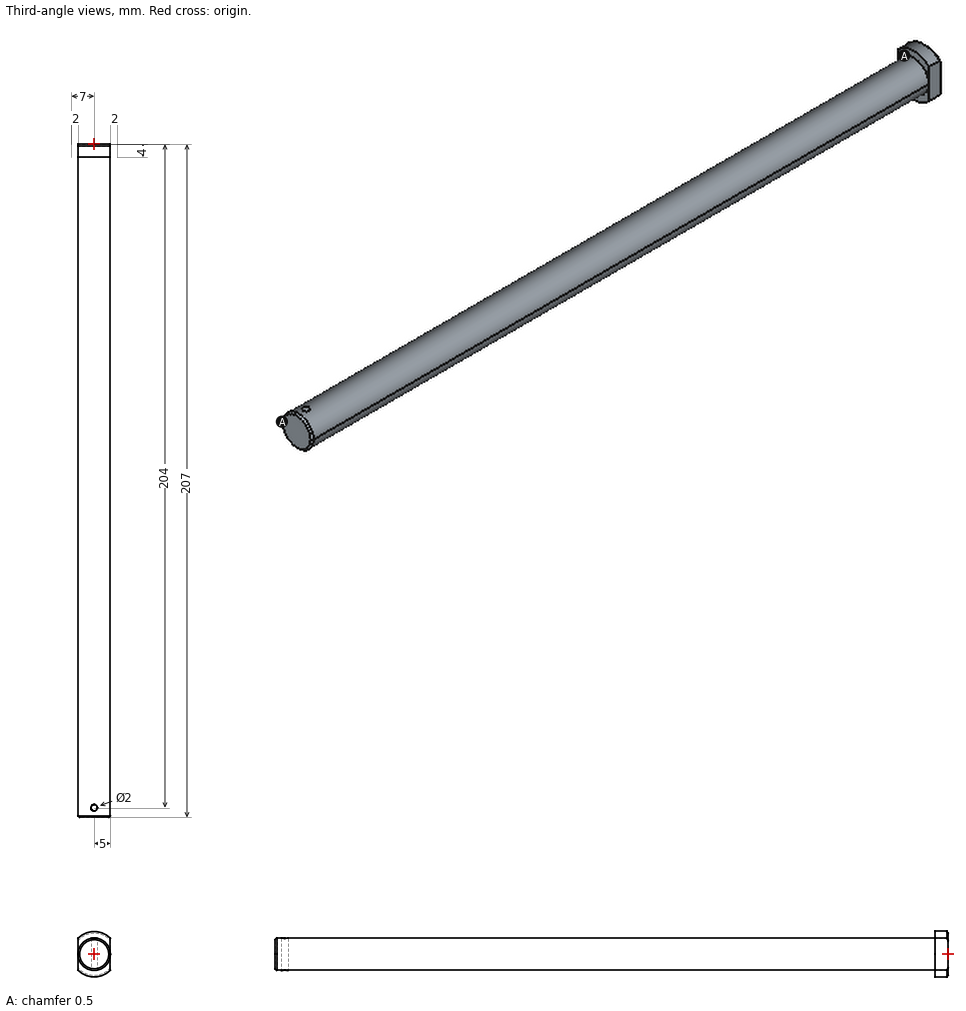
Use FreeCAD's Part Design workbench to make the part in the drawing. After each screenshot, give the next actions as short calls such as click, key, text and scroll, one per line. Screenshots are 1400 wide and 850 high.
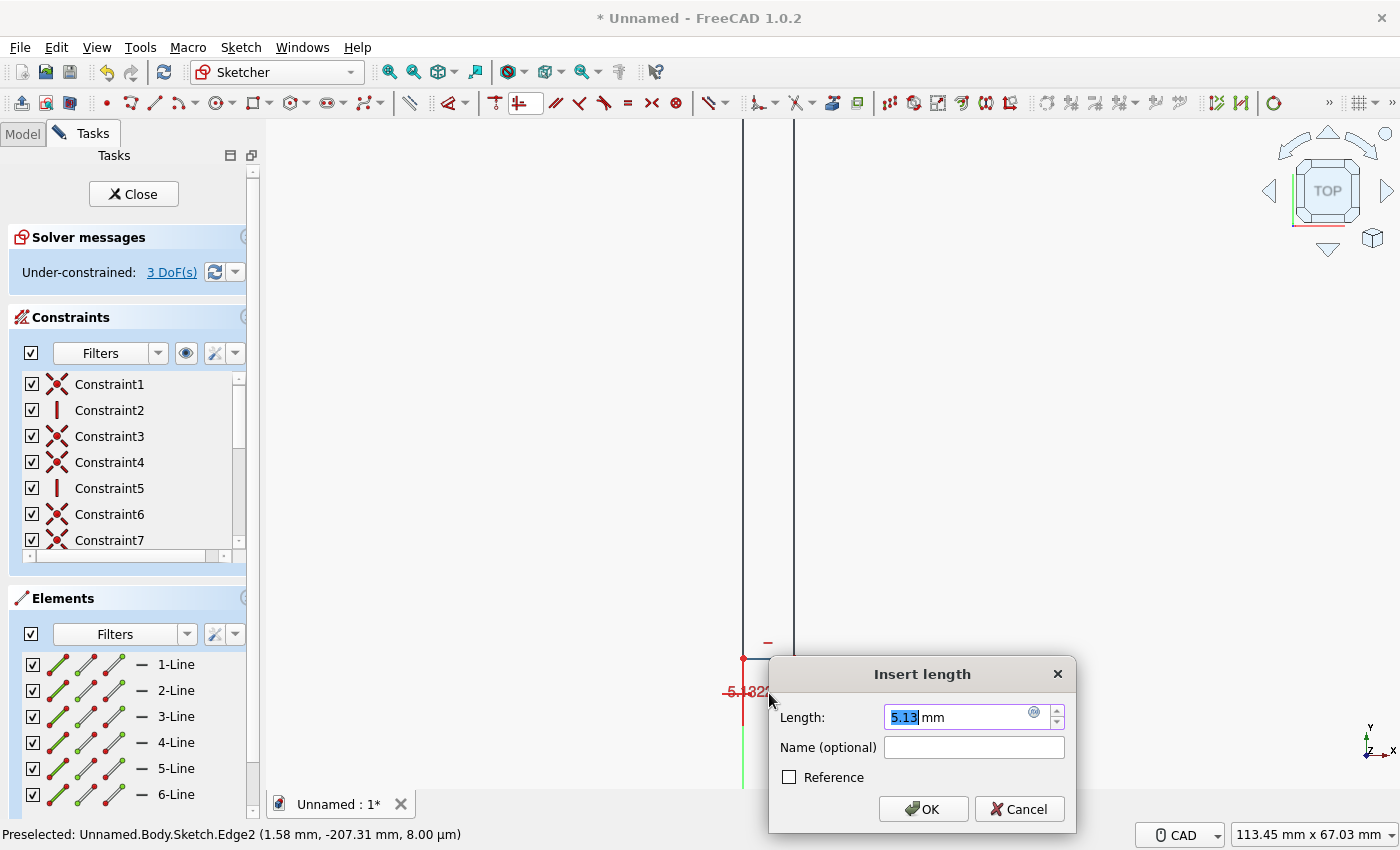
text(5)
key(Return)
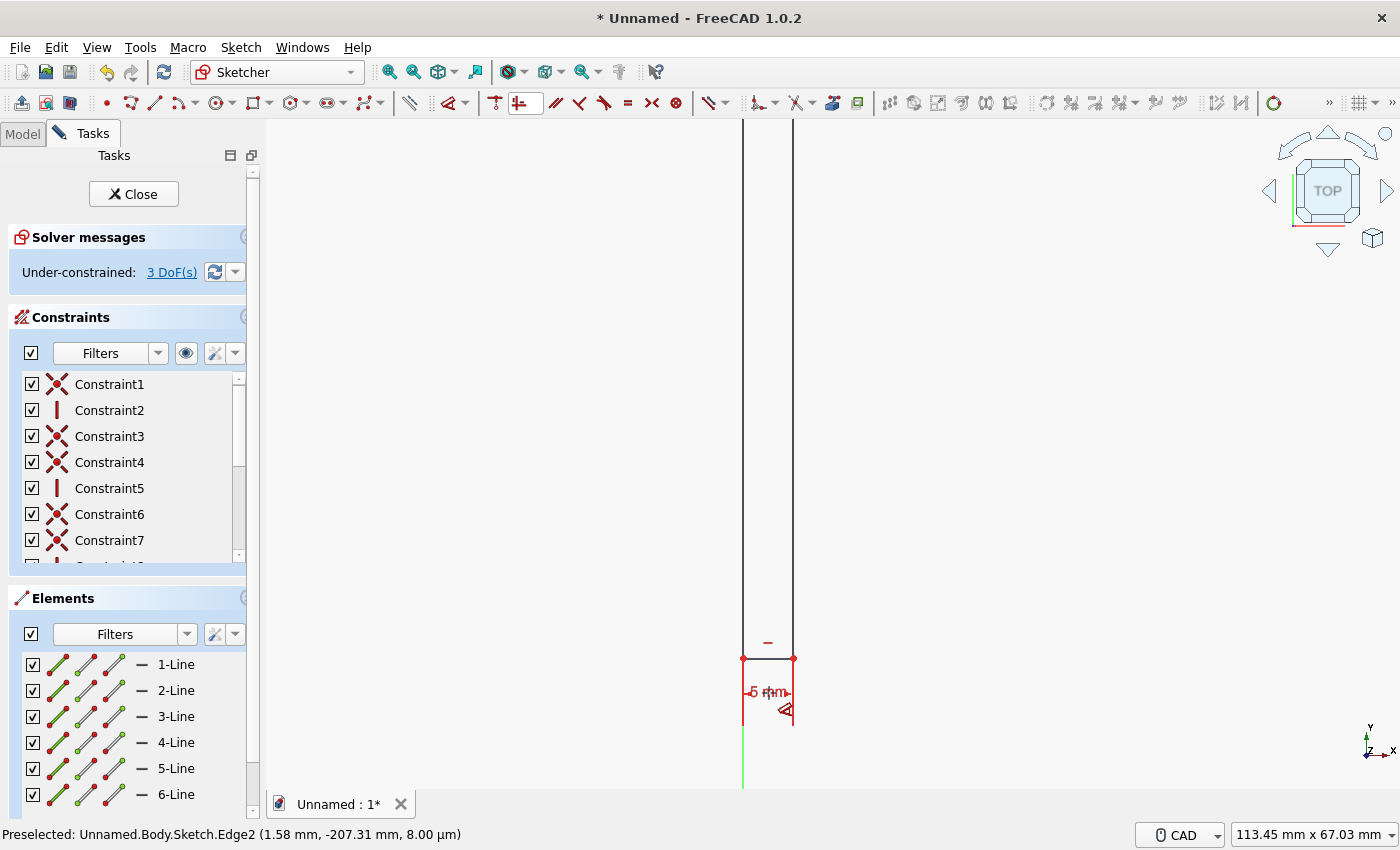
scroll(761, 665, down, 8)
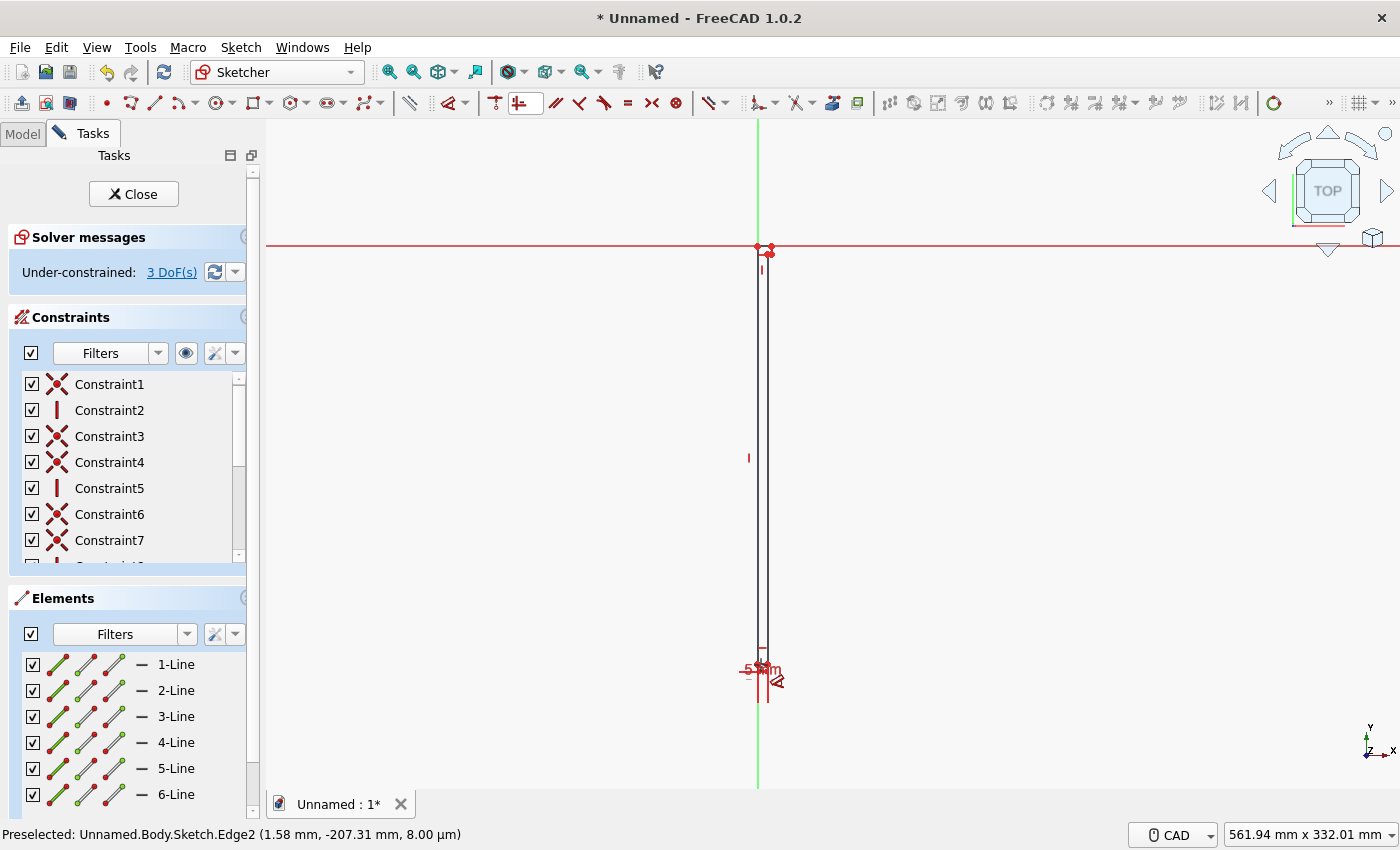
scroll(770, 255, up, 12)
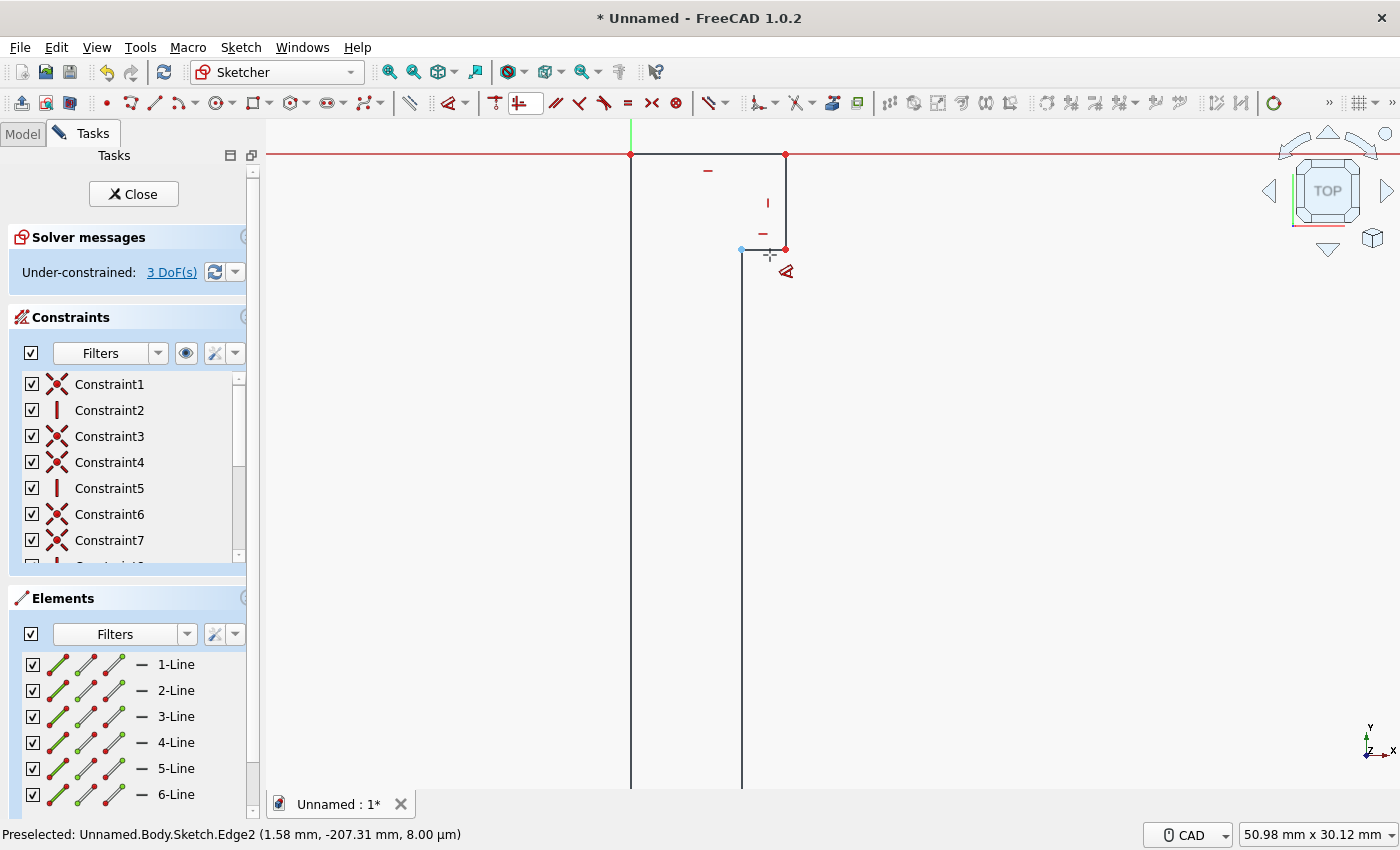
click(764, 250)
click(764, 216)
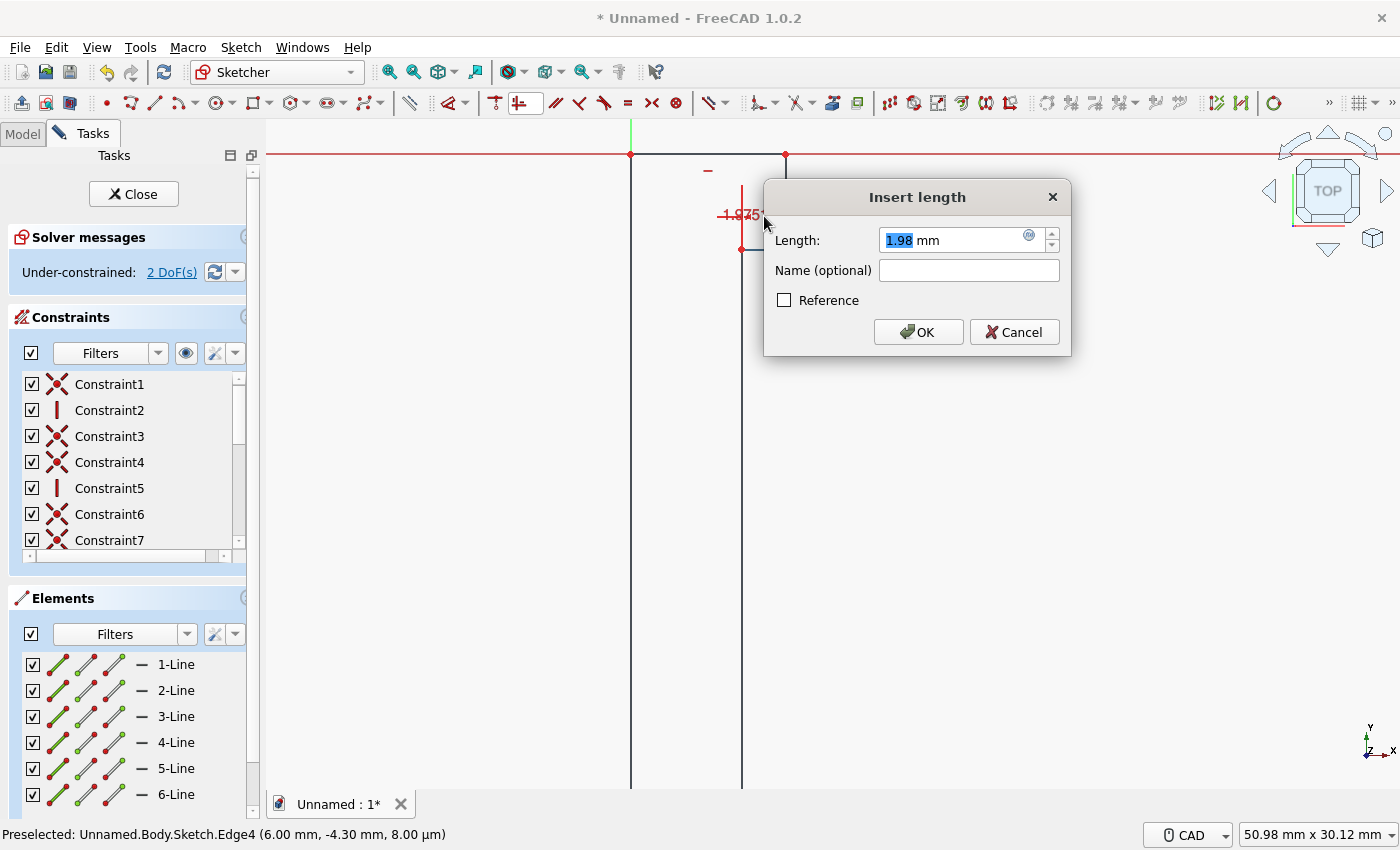
text(2)
key(Return)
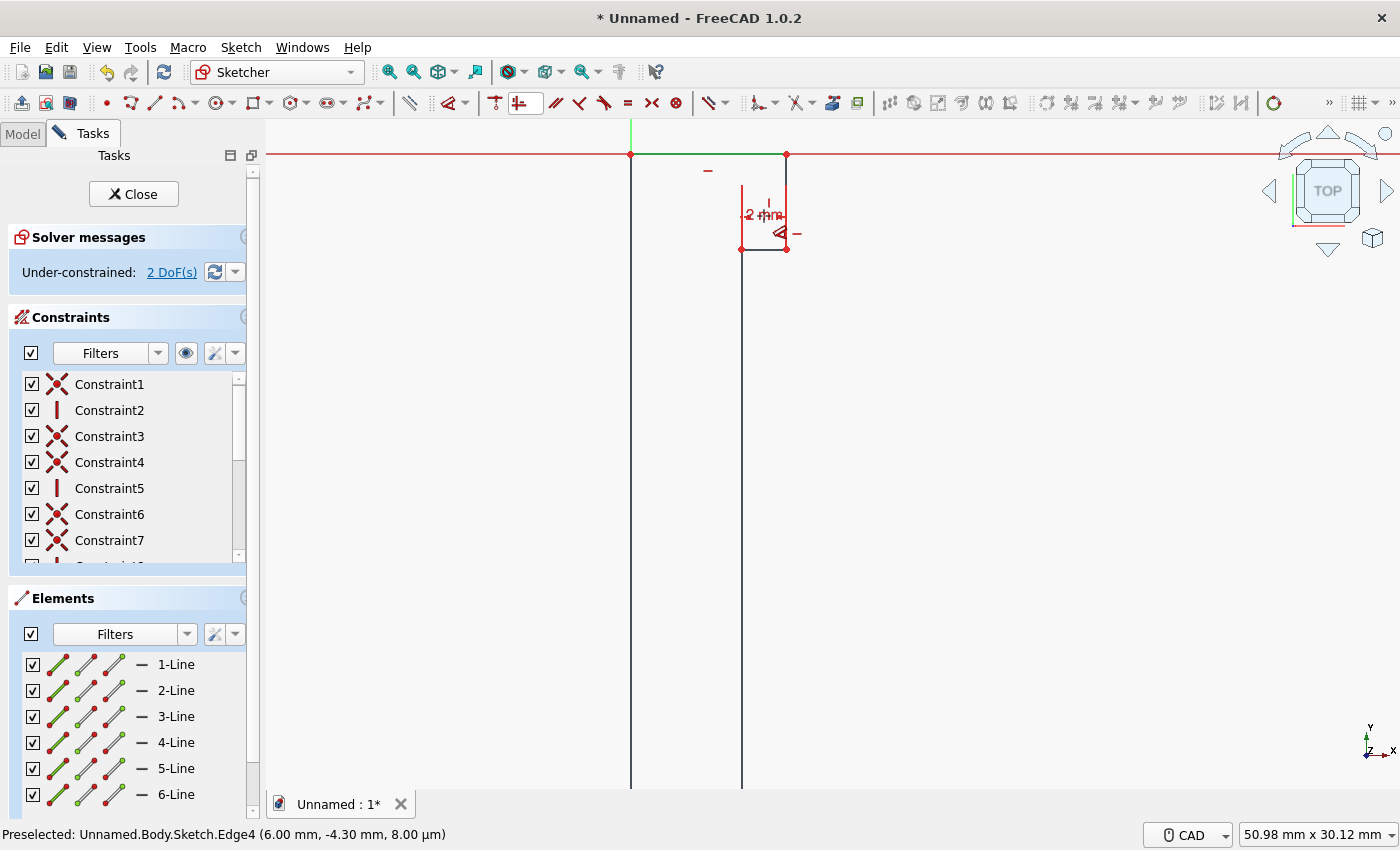
click(786, 221)
click(820, 180)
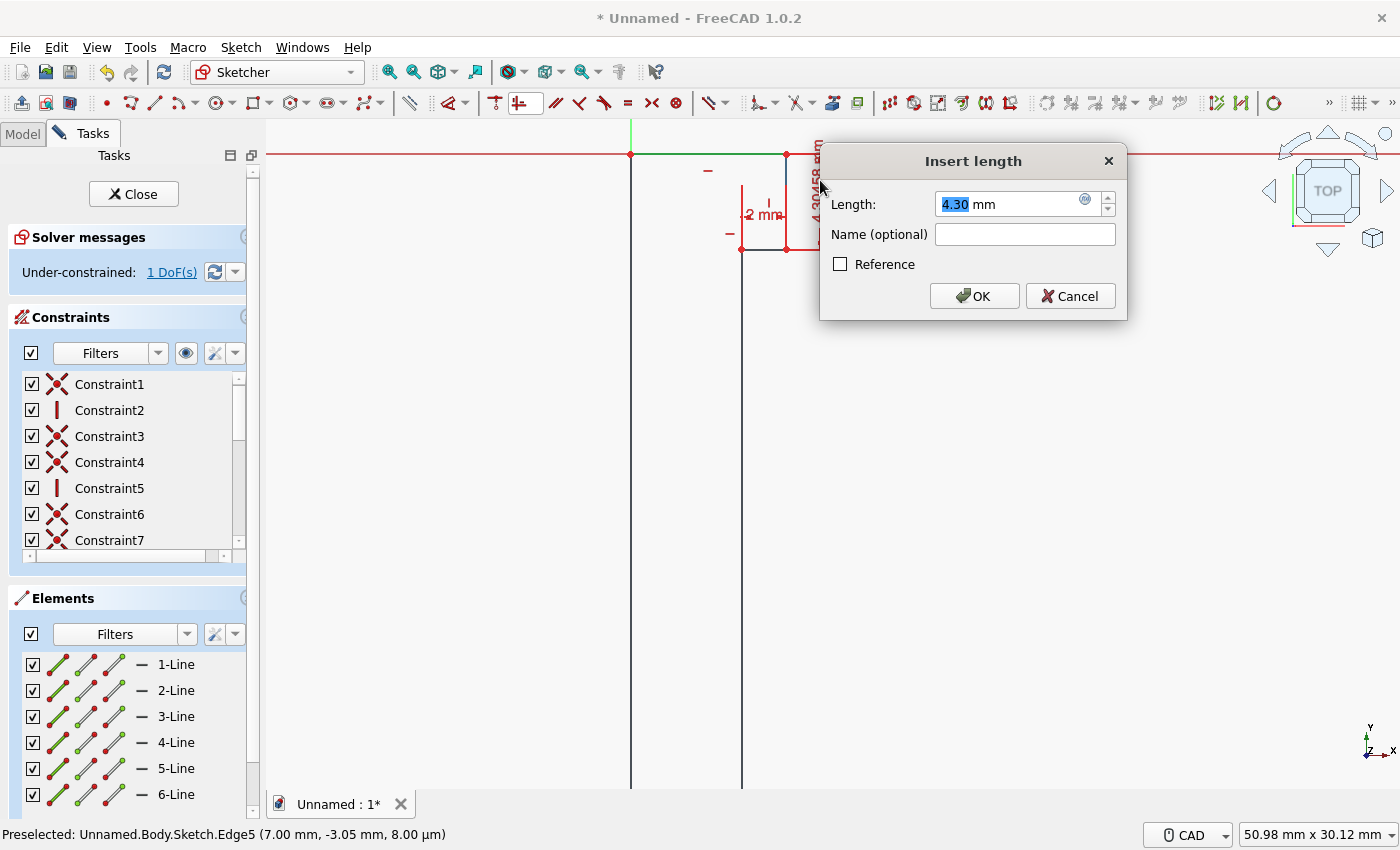
text(4)
key(Return)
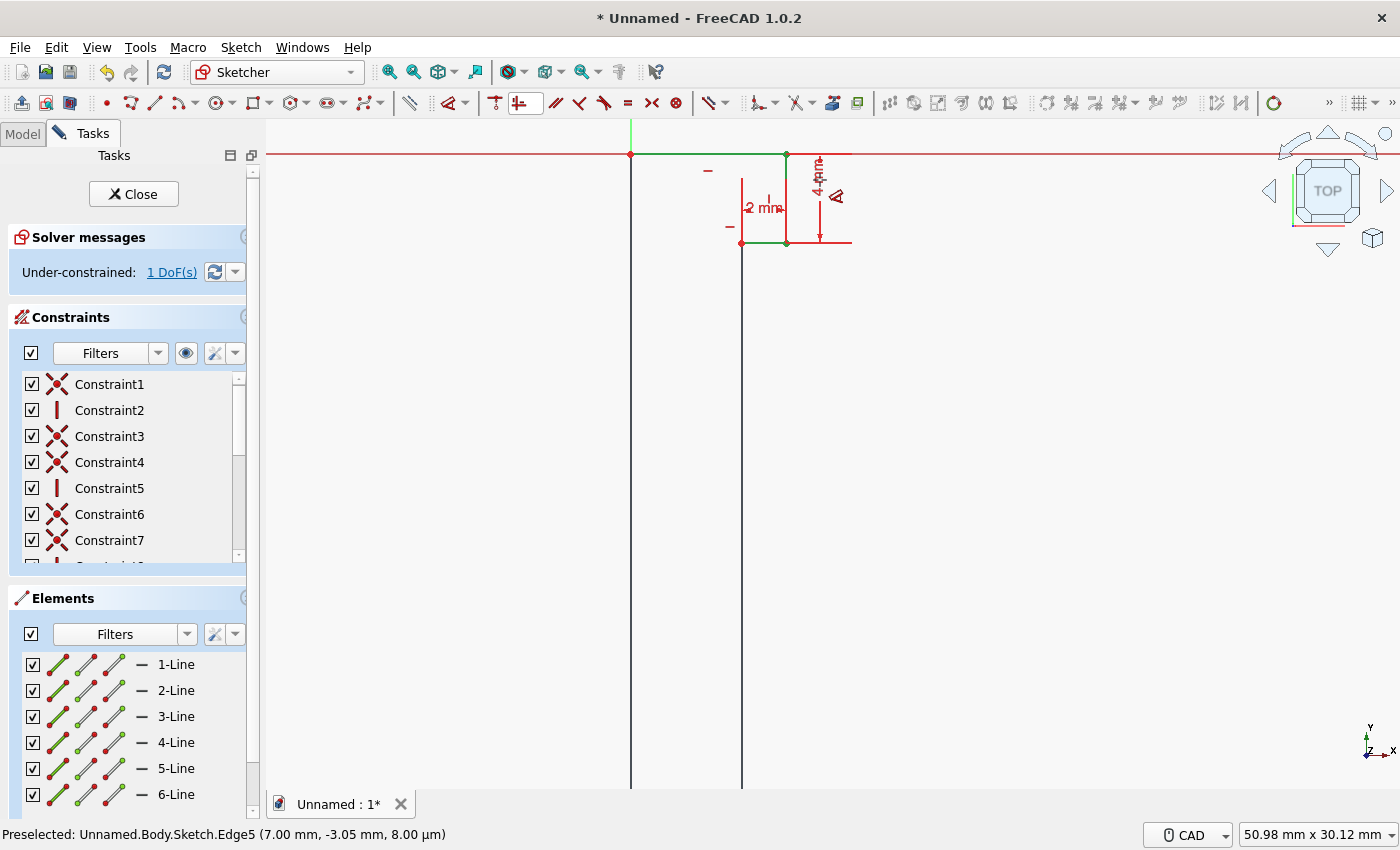
scroll(770, 254, down, 12)